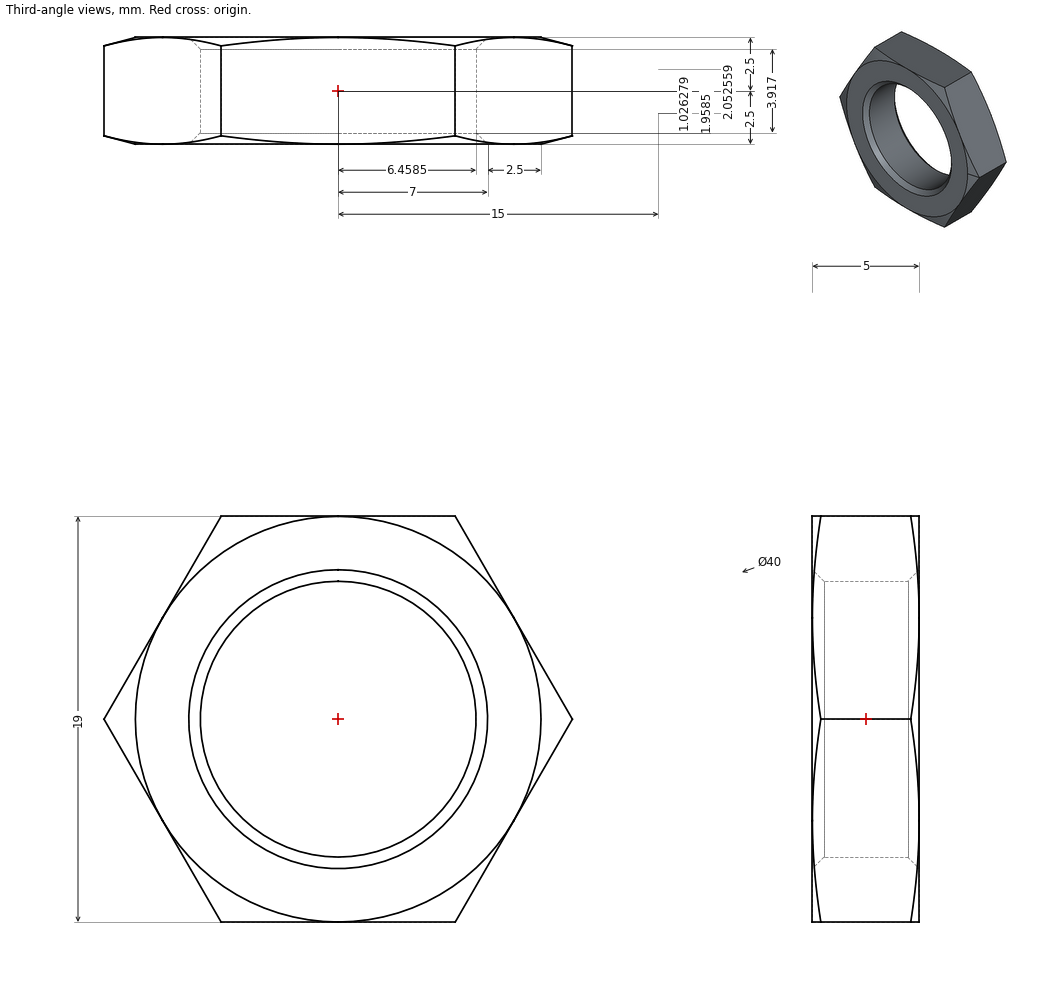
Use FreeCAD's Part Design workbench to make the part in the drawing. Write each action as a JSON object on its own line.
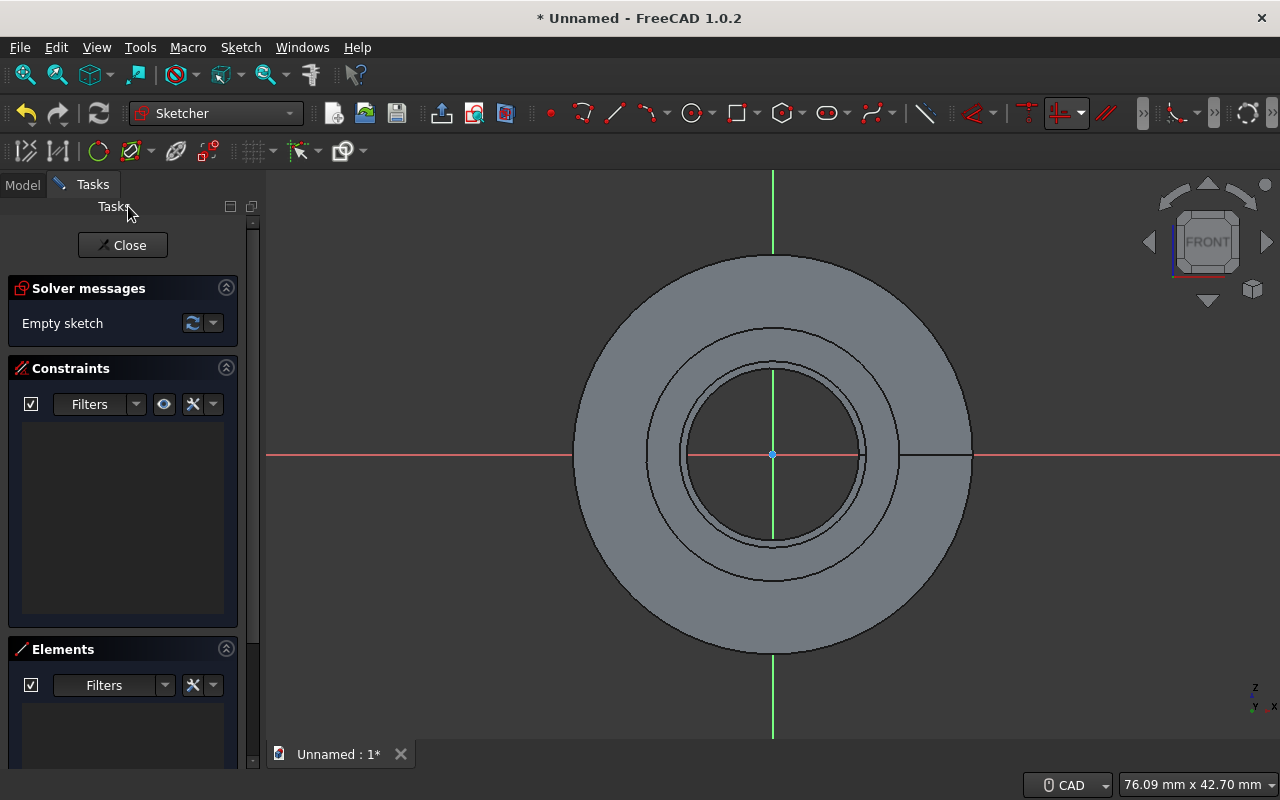
{"action": "left_click", "coordinate": [506, 114]}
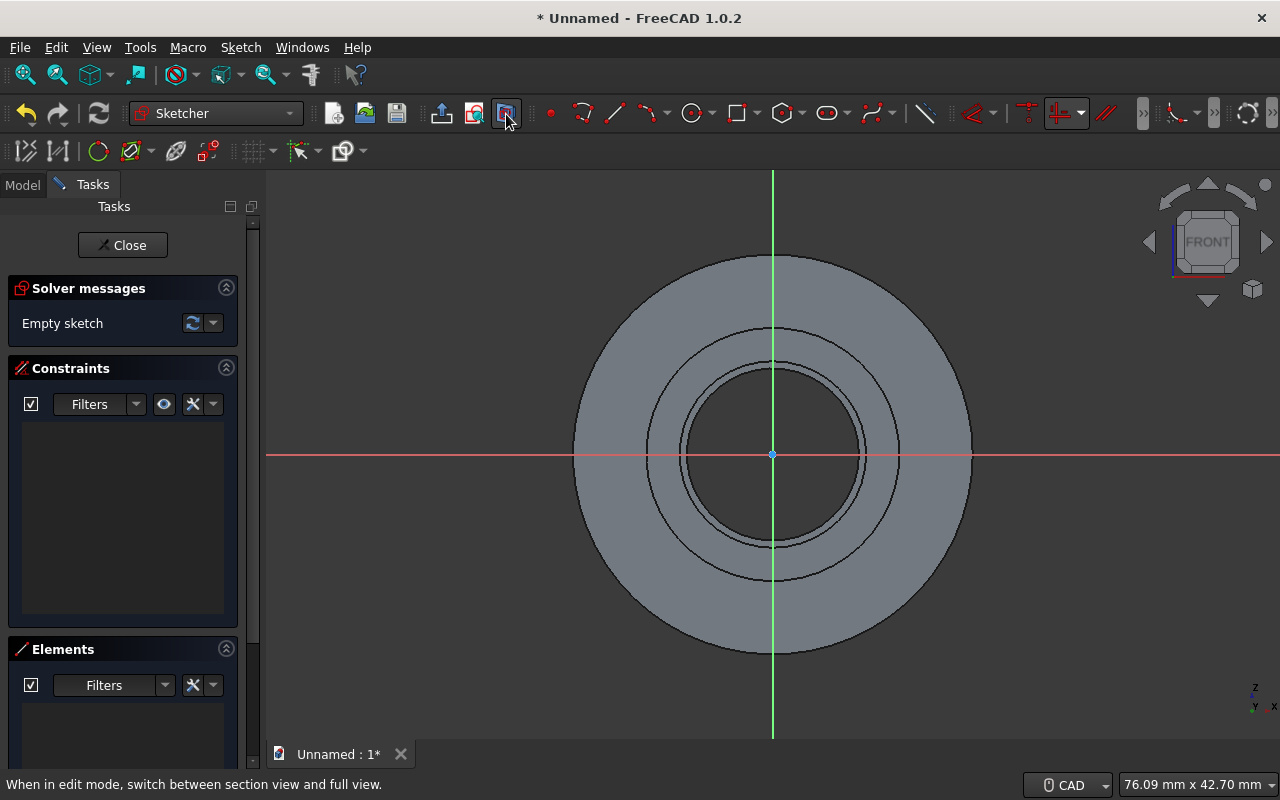
{"action": "scroll", "coordinate": [566, 454], "scroll_direction": "down", "scroll_amount": 2}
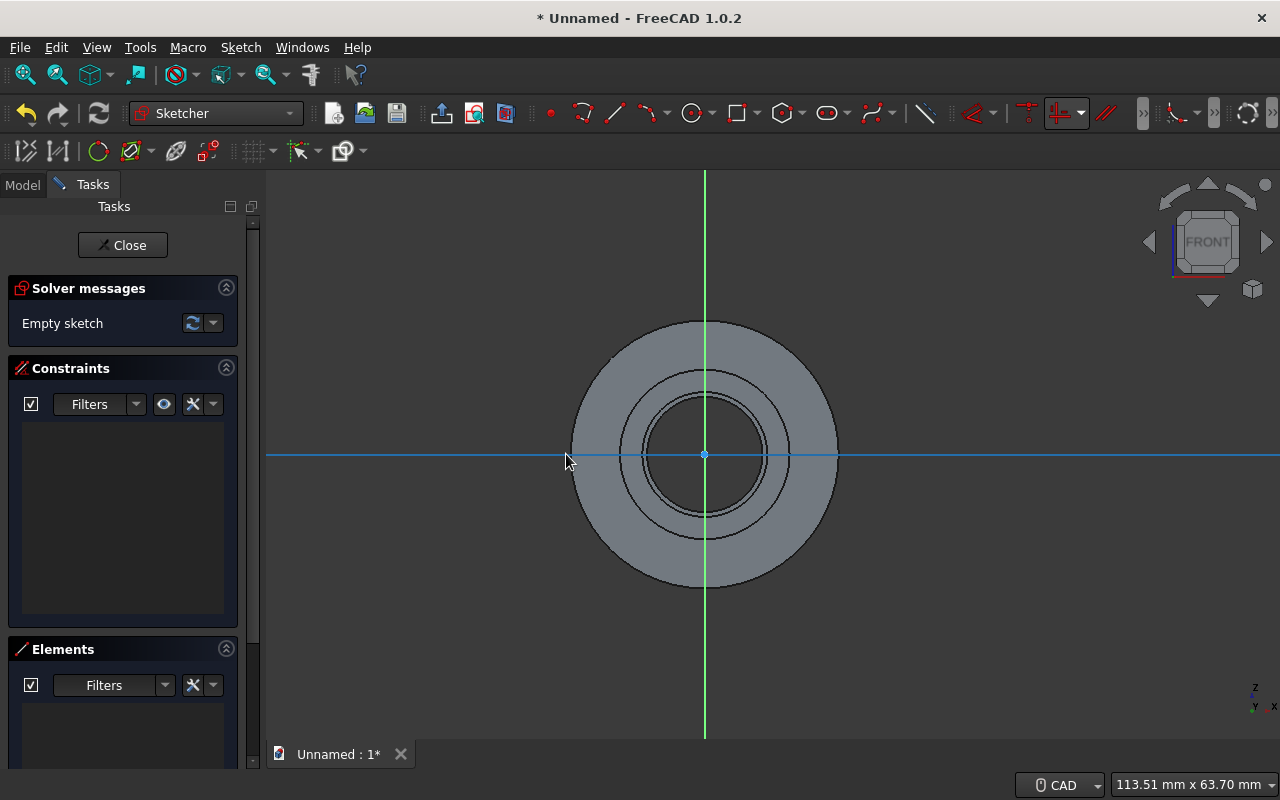
{"action": "left_click", "coordinate": [782, 114]}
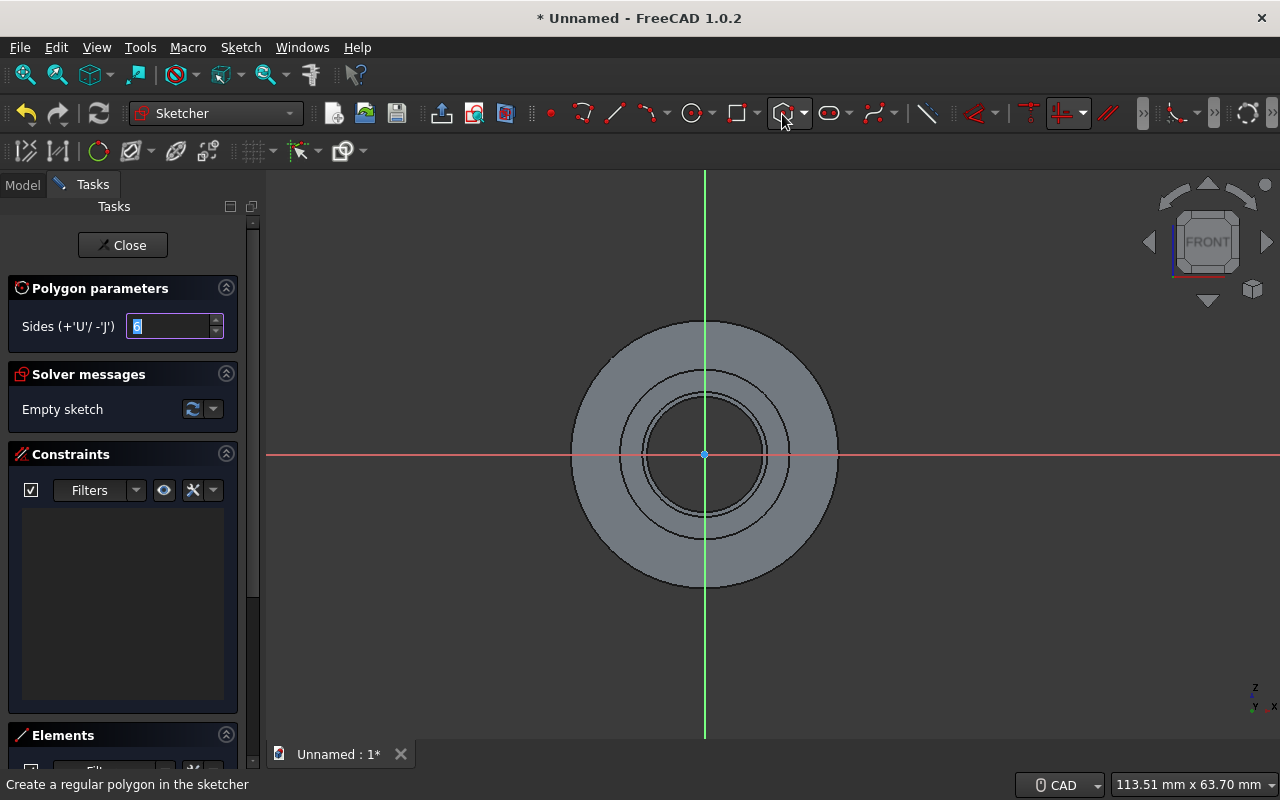
{"action": "left_click", "coordinate": [705, 455]}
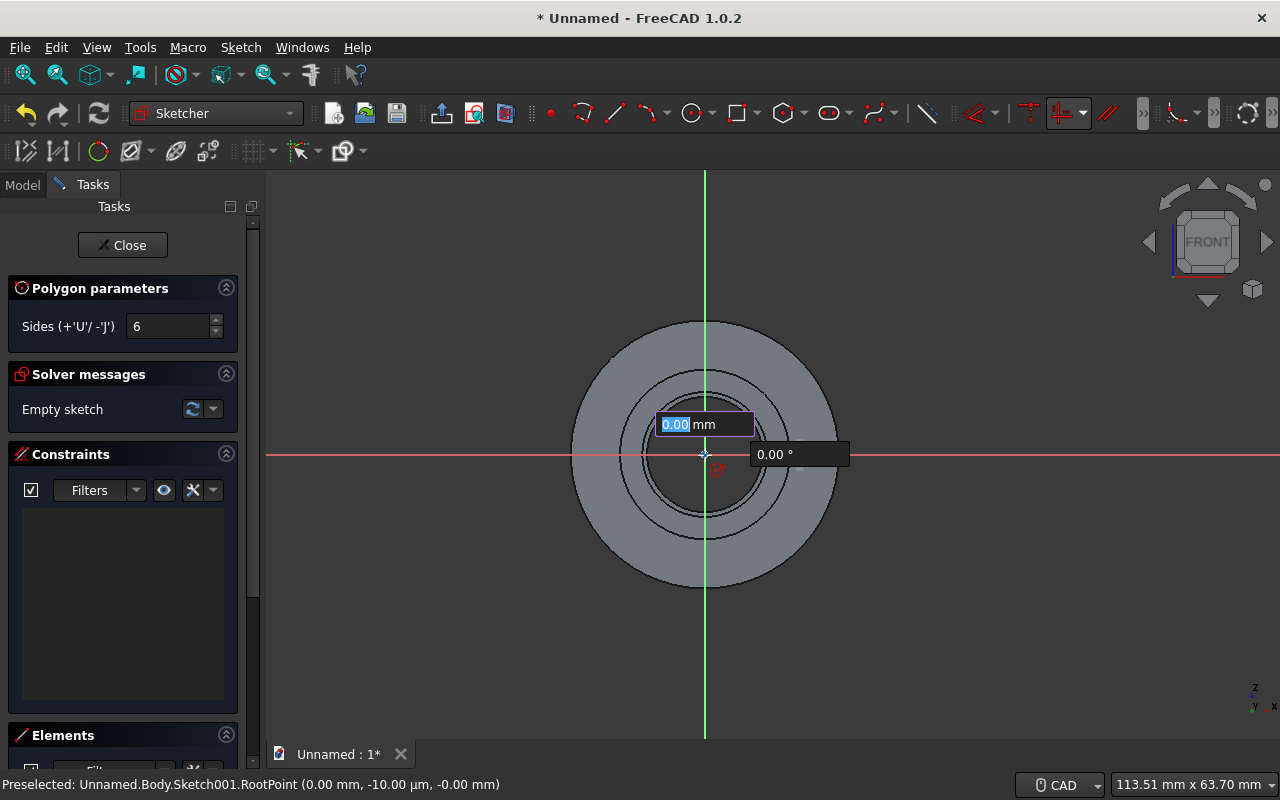
{"action": "left_click", "coordinate": [607, 455]}
{"action": "key", "text": "Escape"}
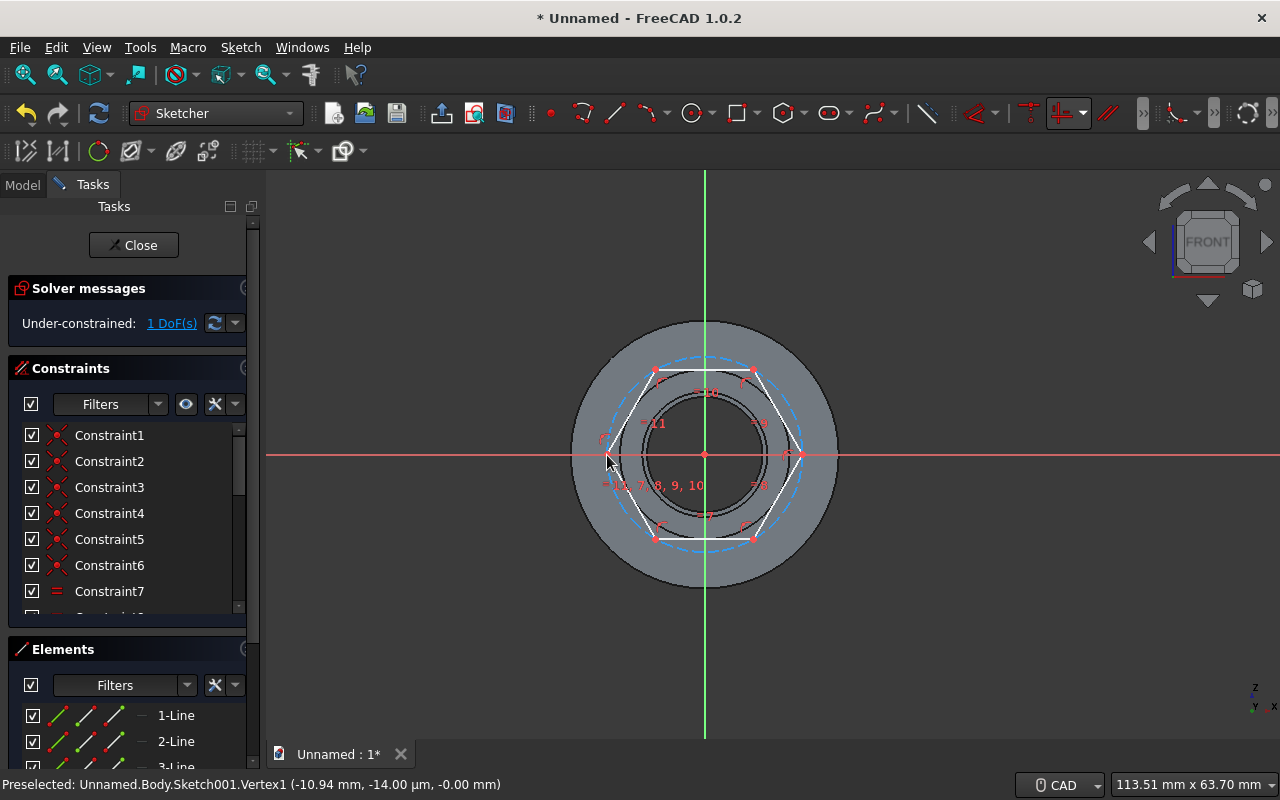
{"action": "left_click", "coordinate": [692, 114]}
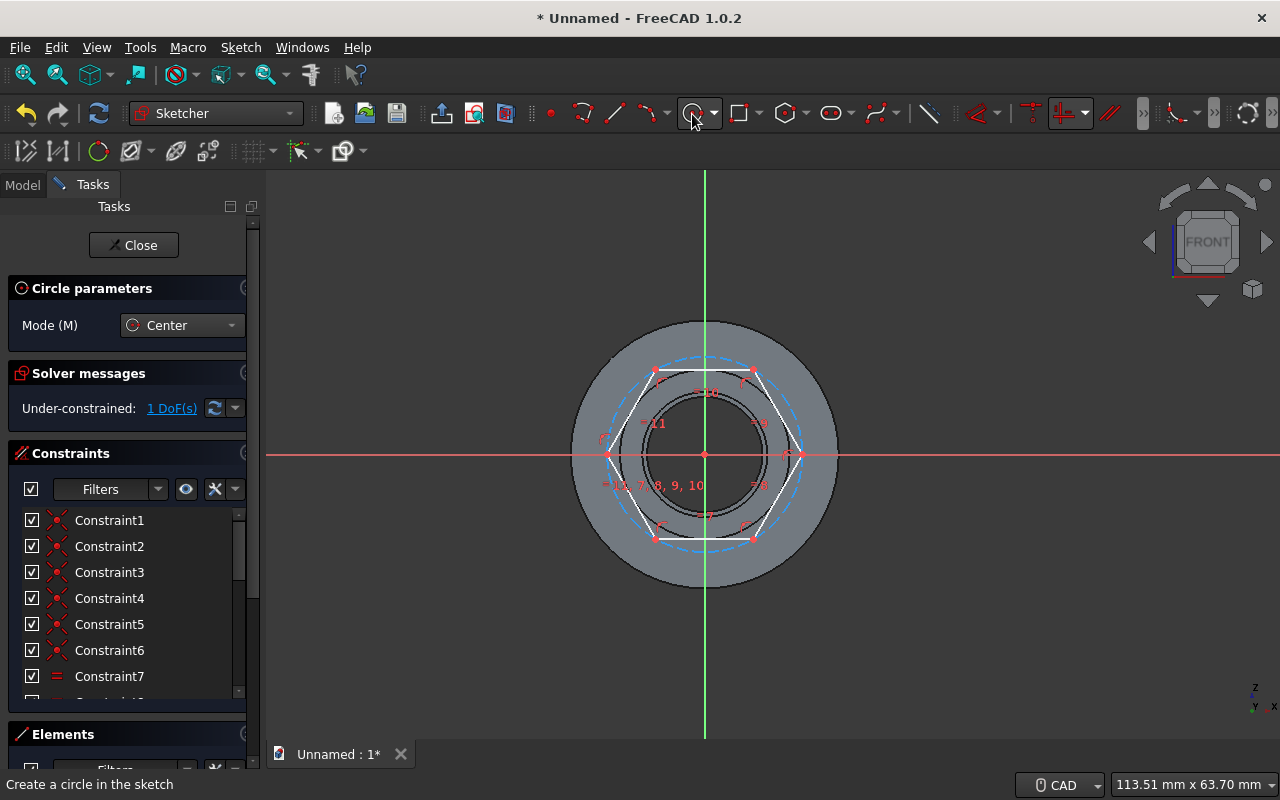
{"action": "left_click", "coordinate": [705, 455]}
{"action": "mouse_move", "coordinate": [831, 328]}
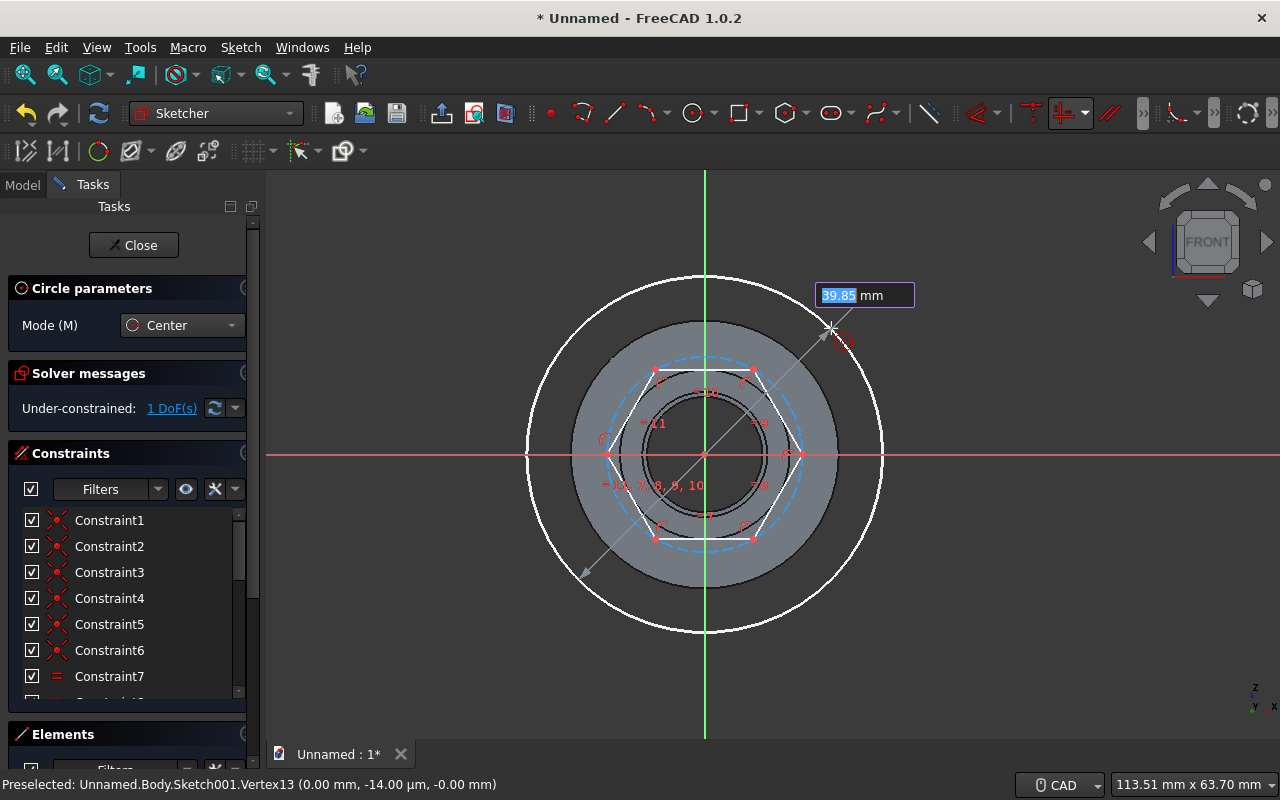
{"action": "type", "text": "40"}
{"action": "key", "text": "Return"}
{"action": "key", "text": "Escape"}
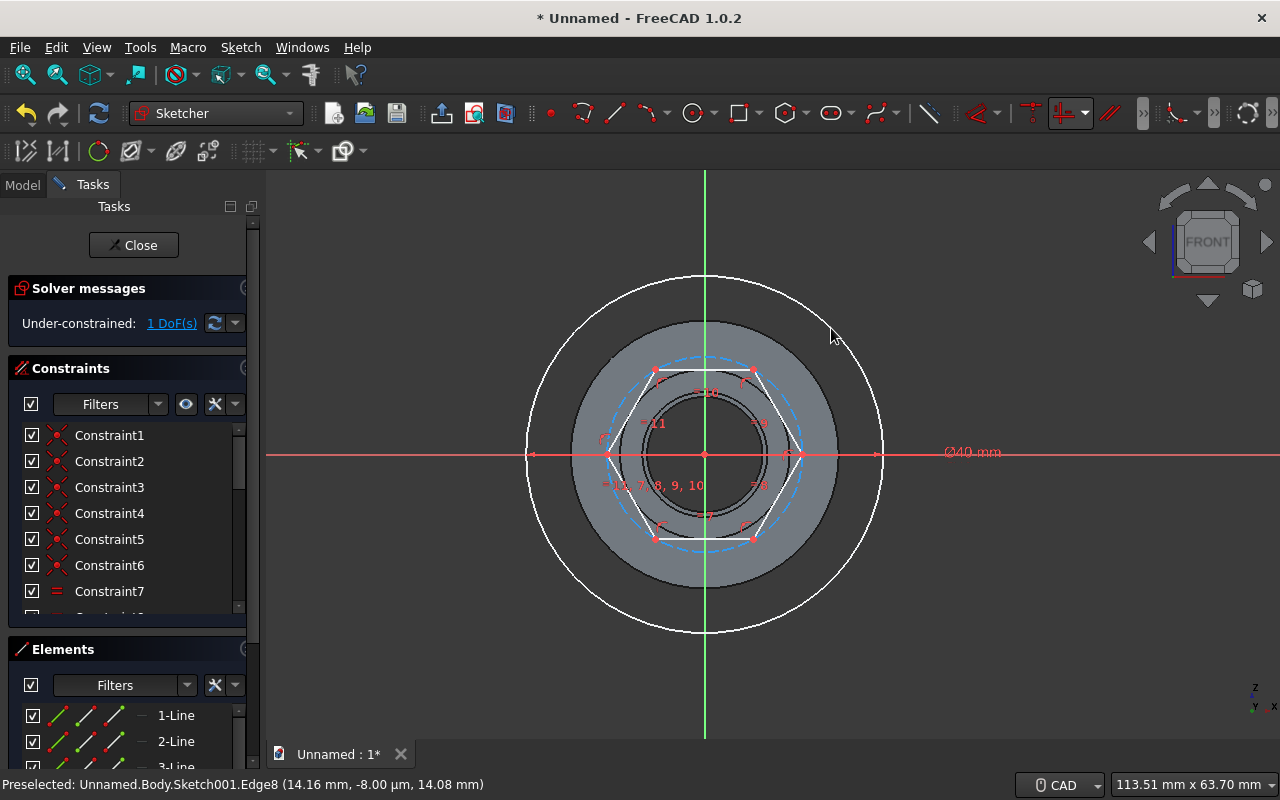
{"action": "key", "text": "d"}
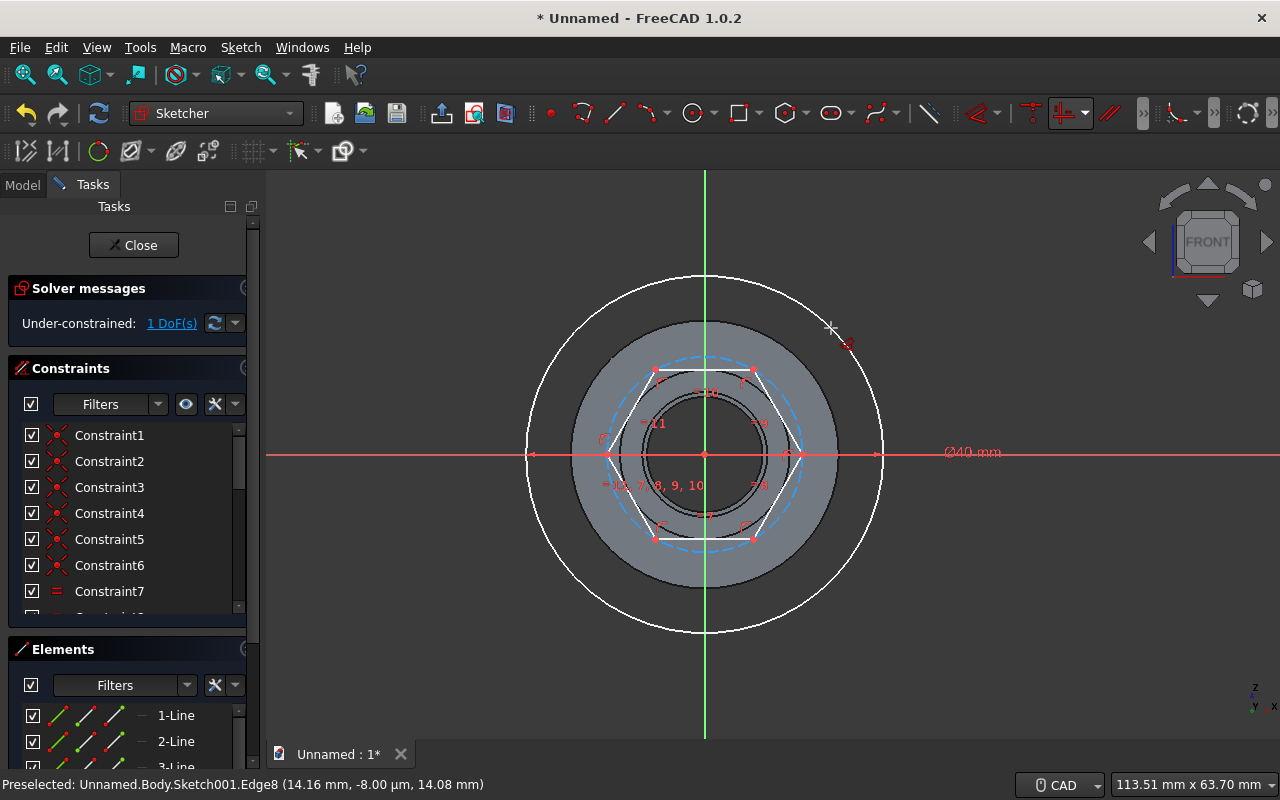
{"action": "left_click", "coordinate": [656, 539]}